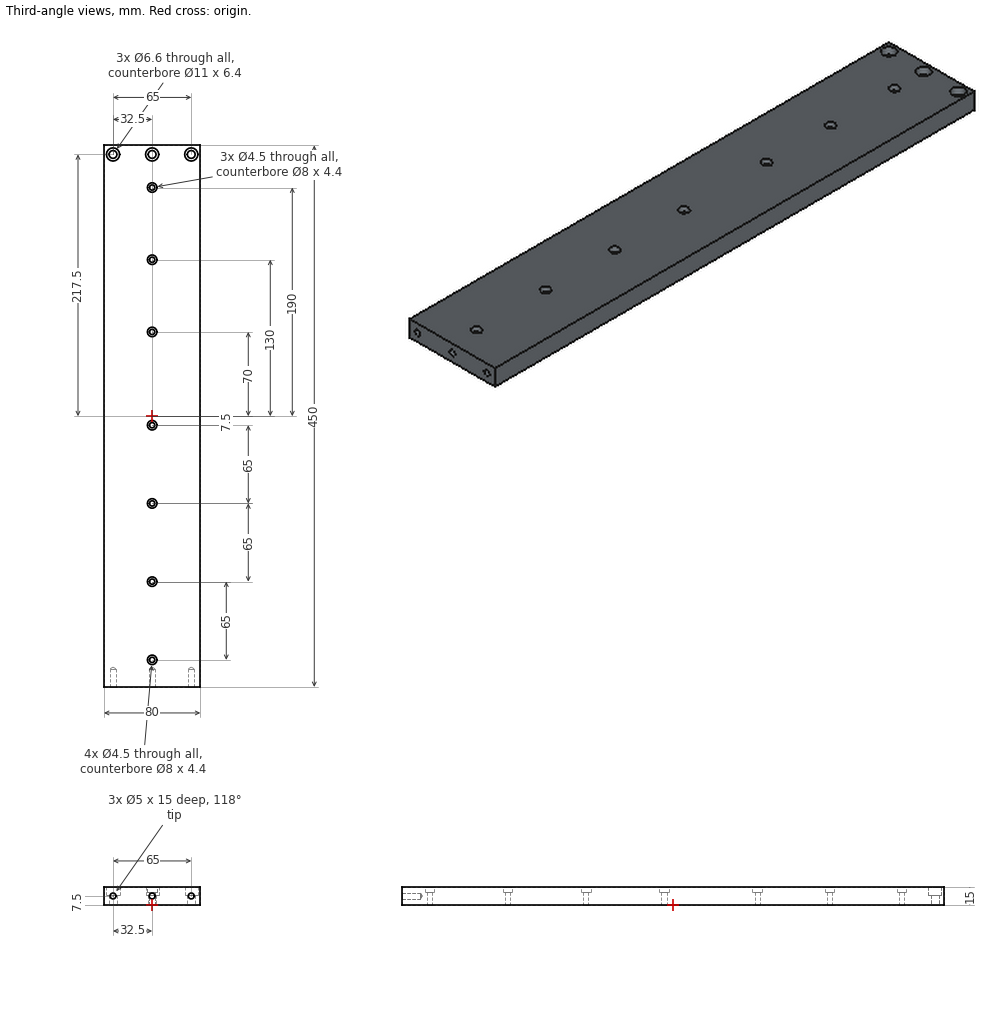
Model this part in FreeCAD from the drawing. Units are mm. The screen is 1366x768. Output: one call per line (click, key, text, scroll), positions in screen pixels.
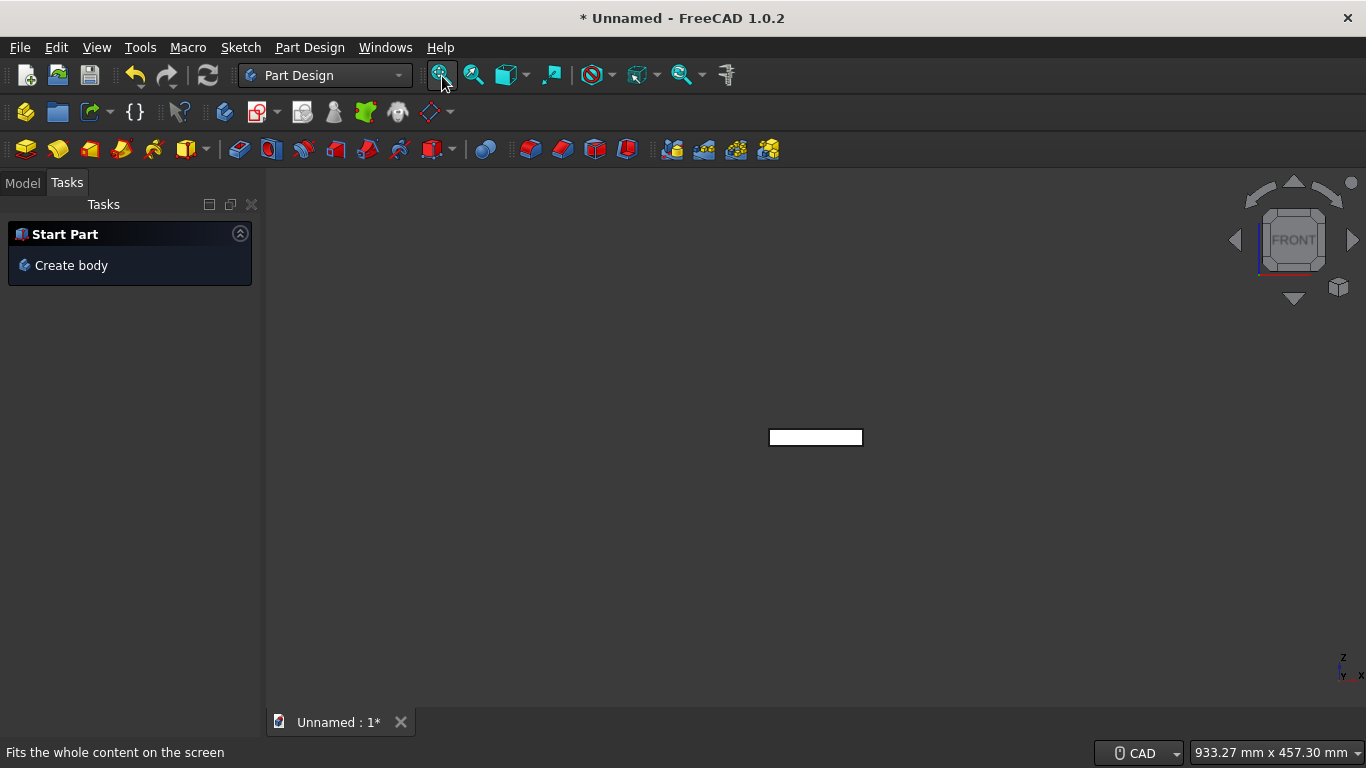
click(843, 437)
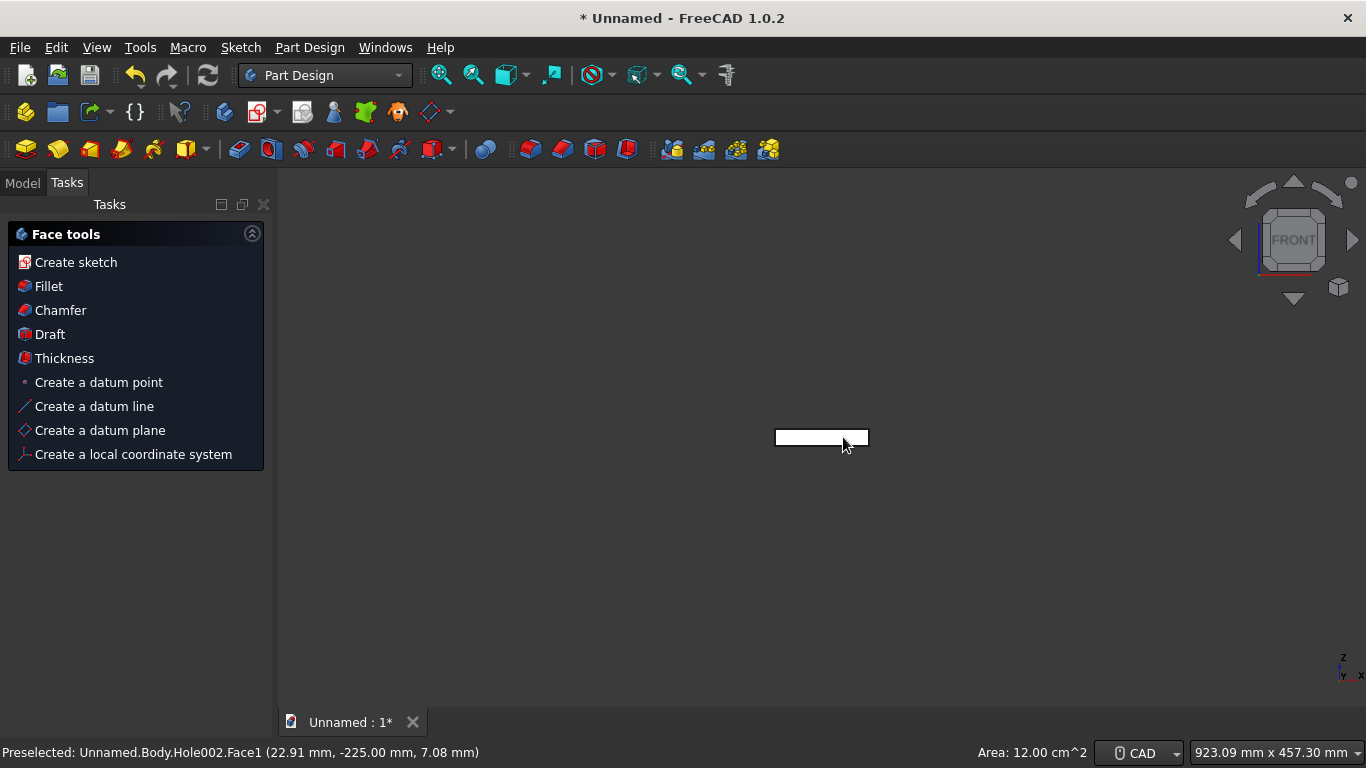
click(258, 112)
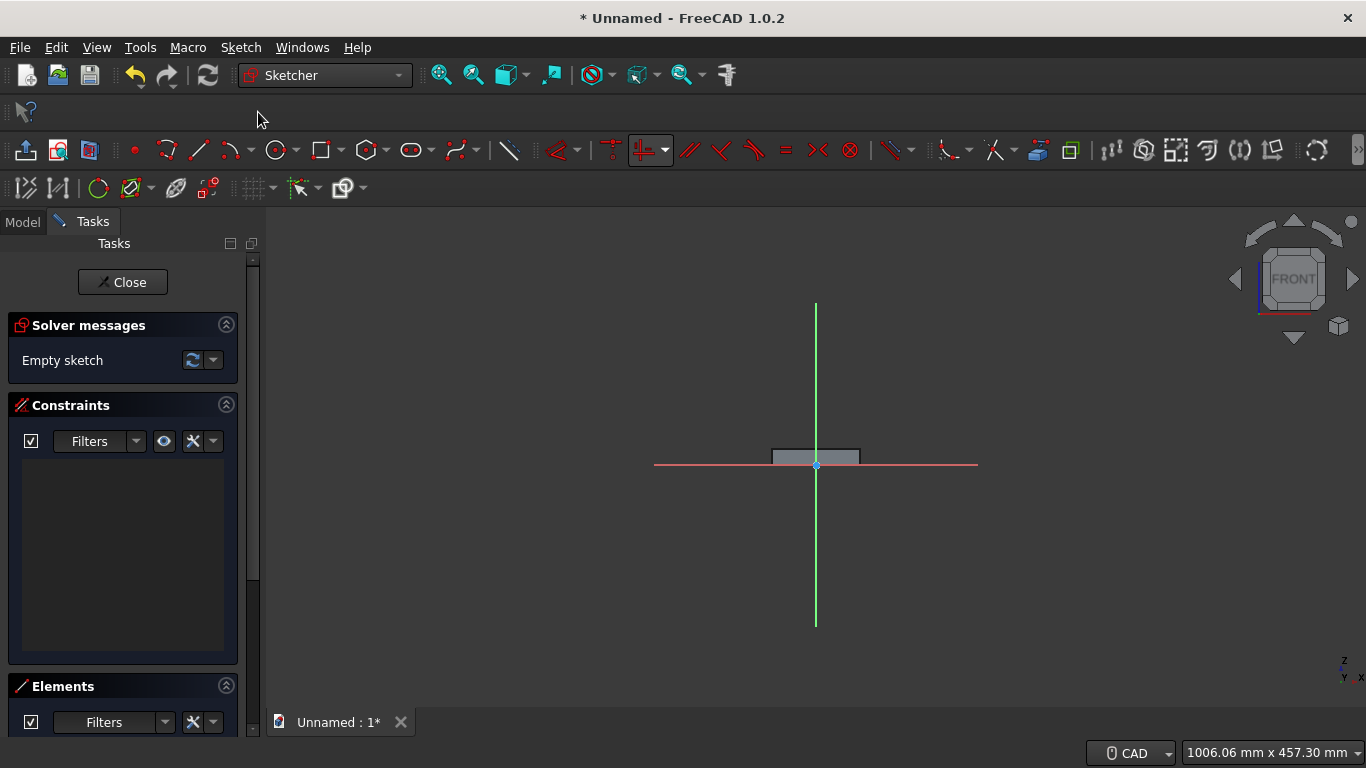
scroll(825, 460, up, 11)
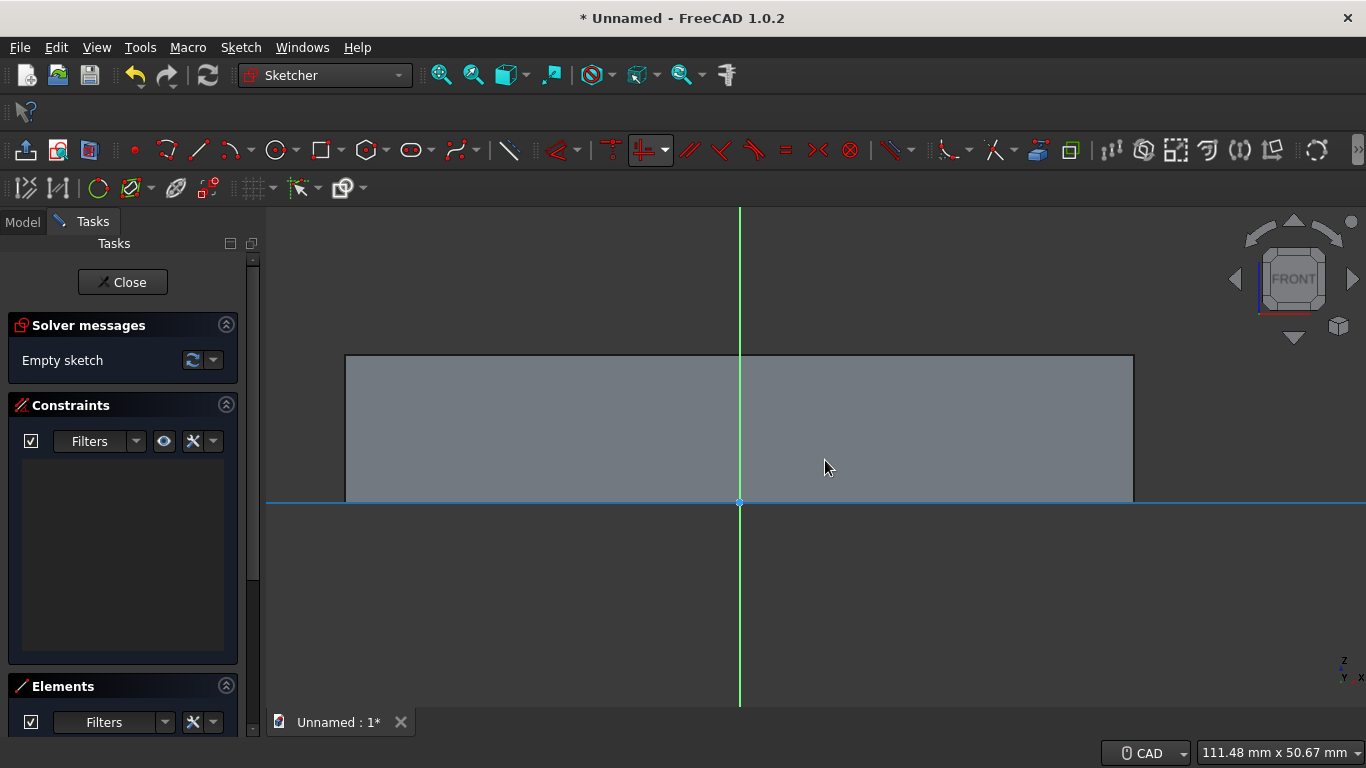
click(276, 150)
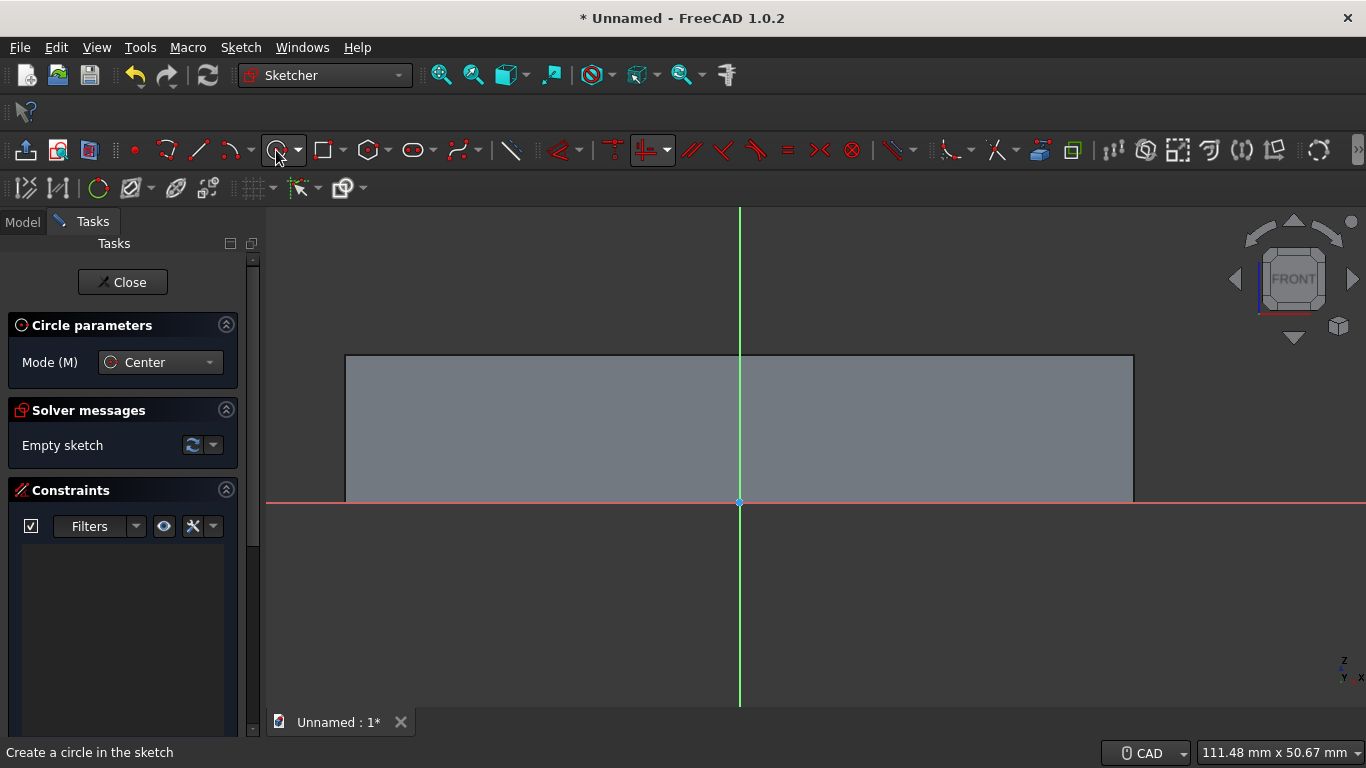
click(419, 429)
move(436, 411)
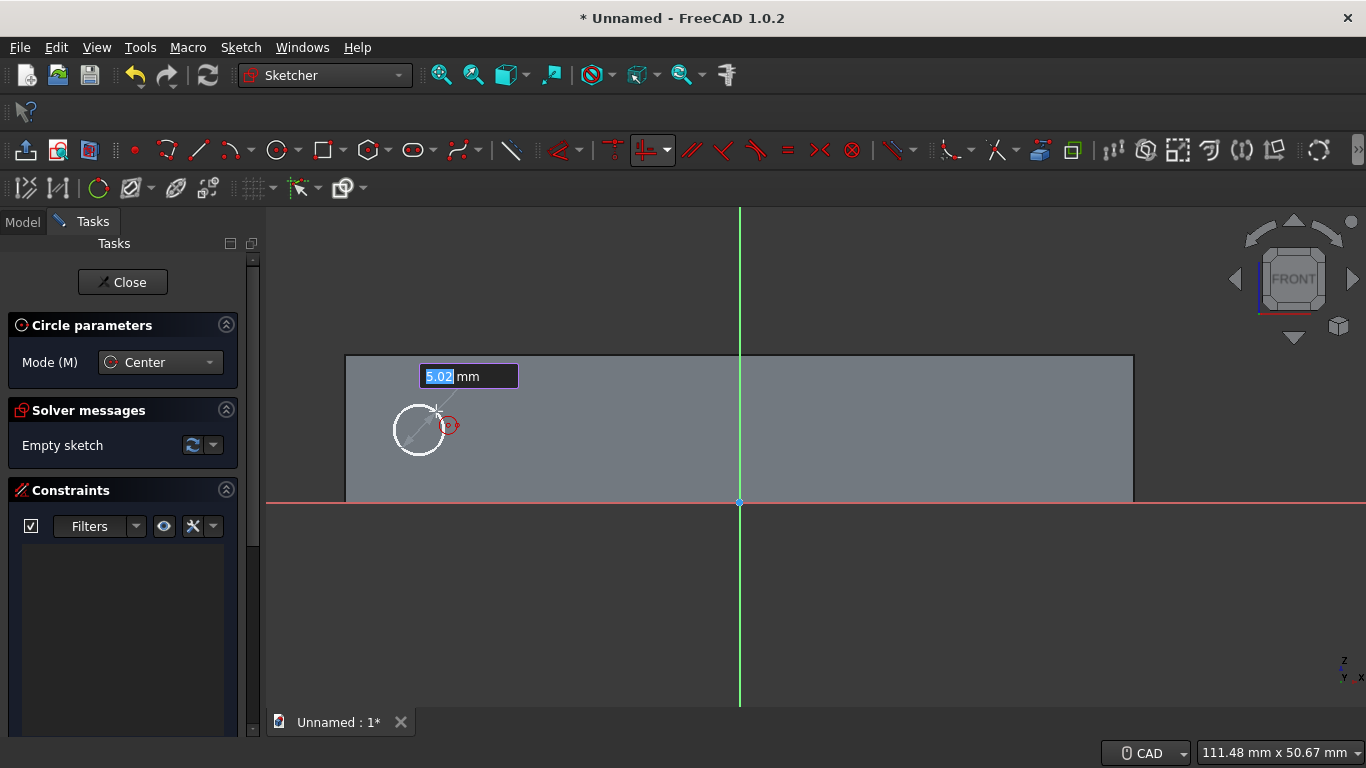
text(5)
key(Return)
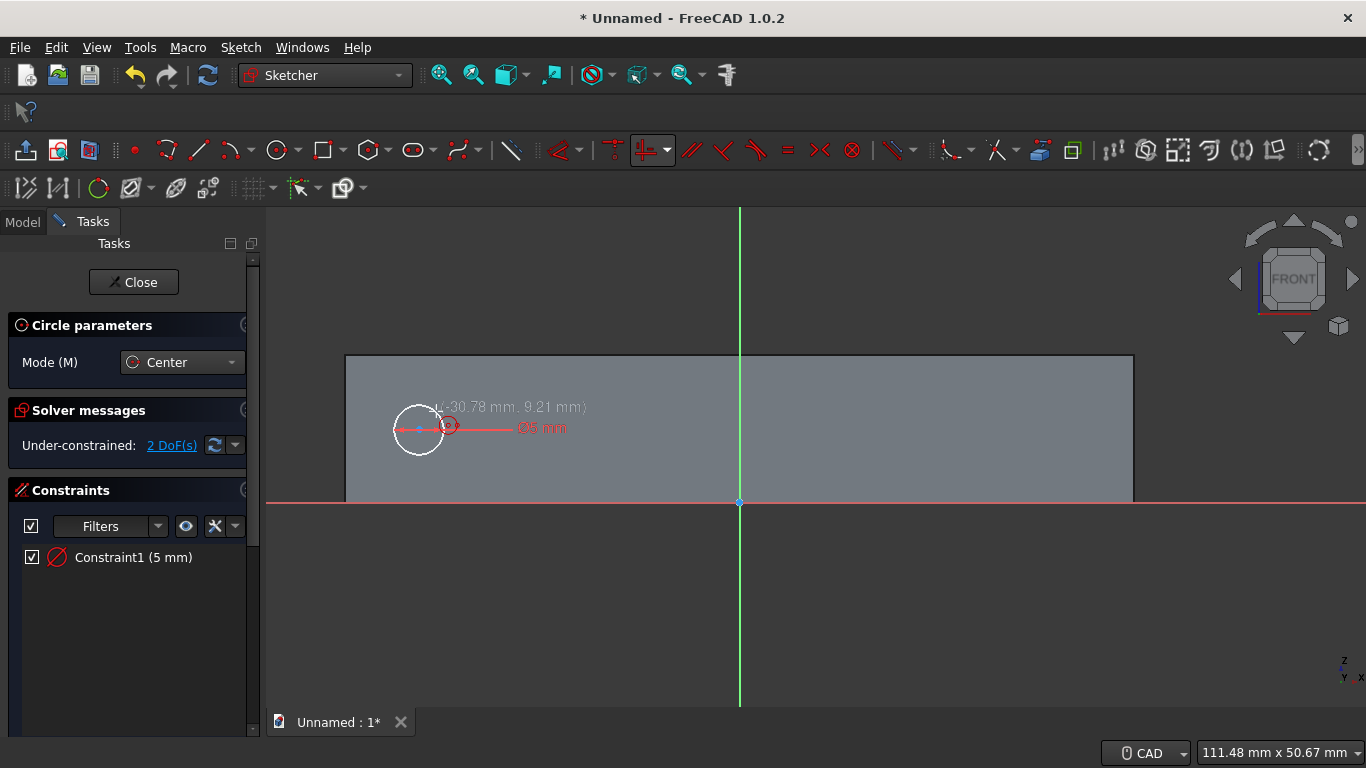
click(740, 429)
move(757, 411)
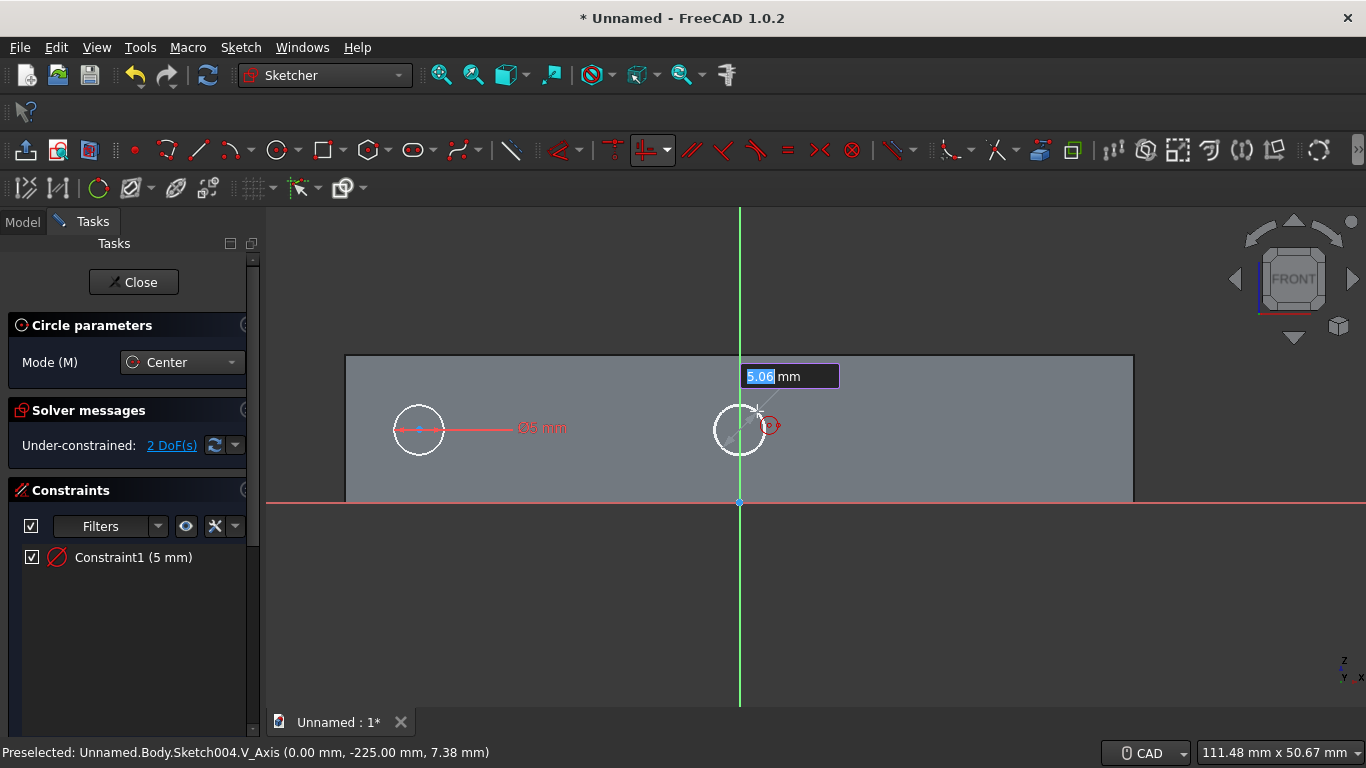
text(5)
key(Return)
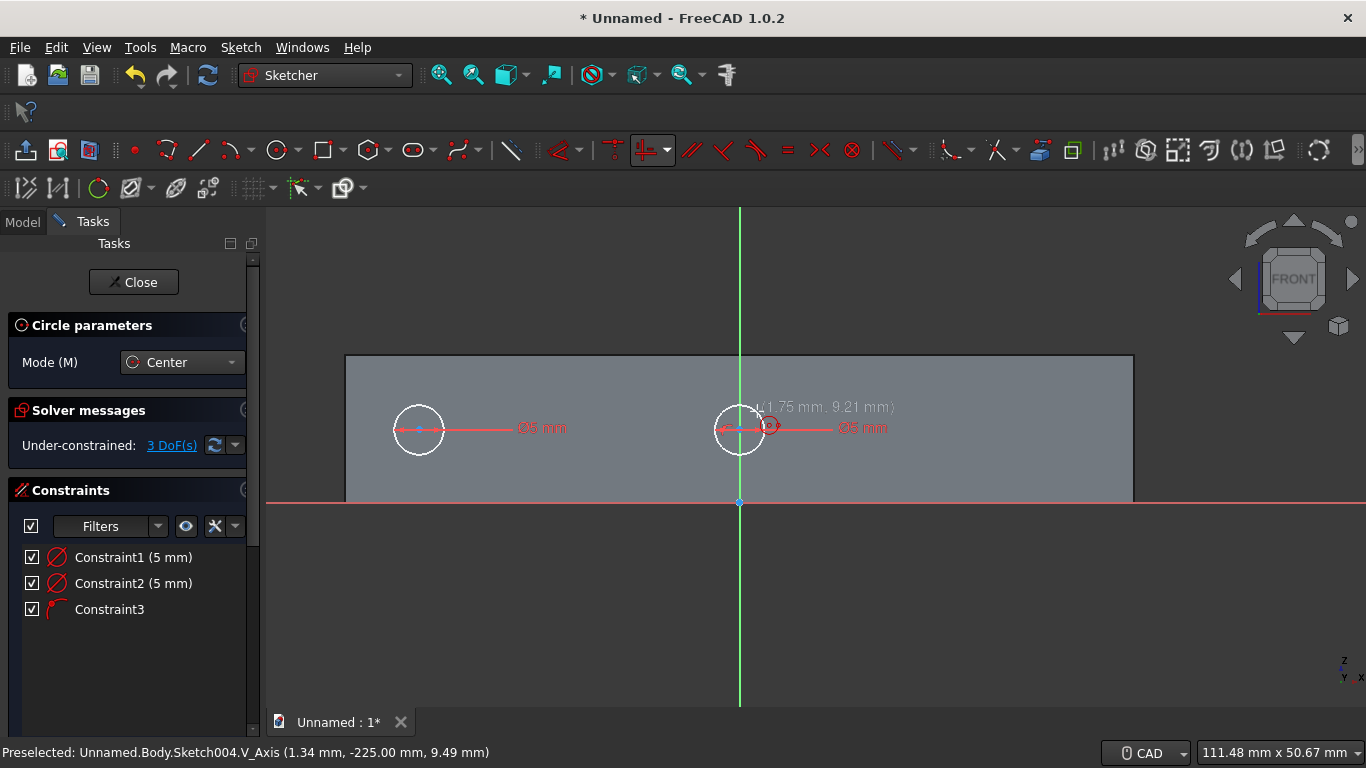
click(1060, 429)
move(1078, 411)